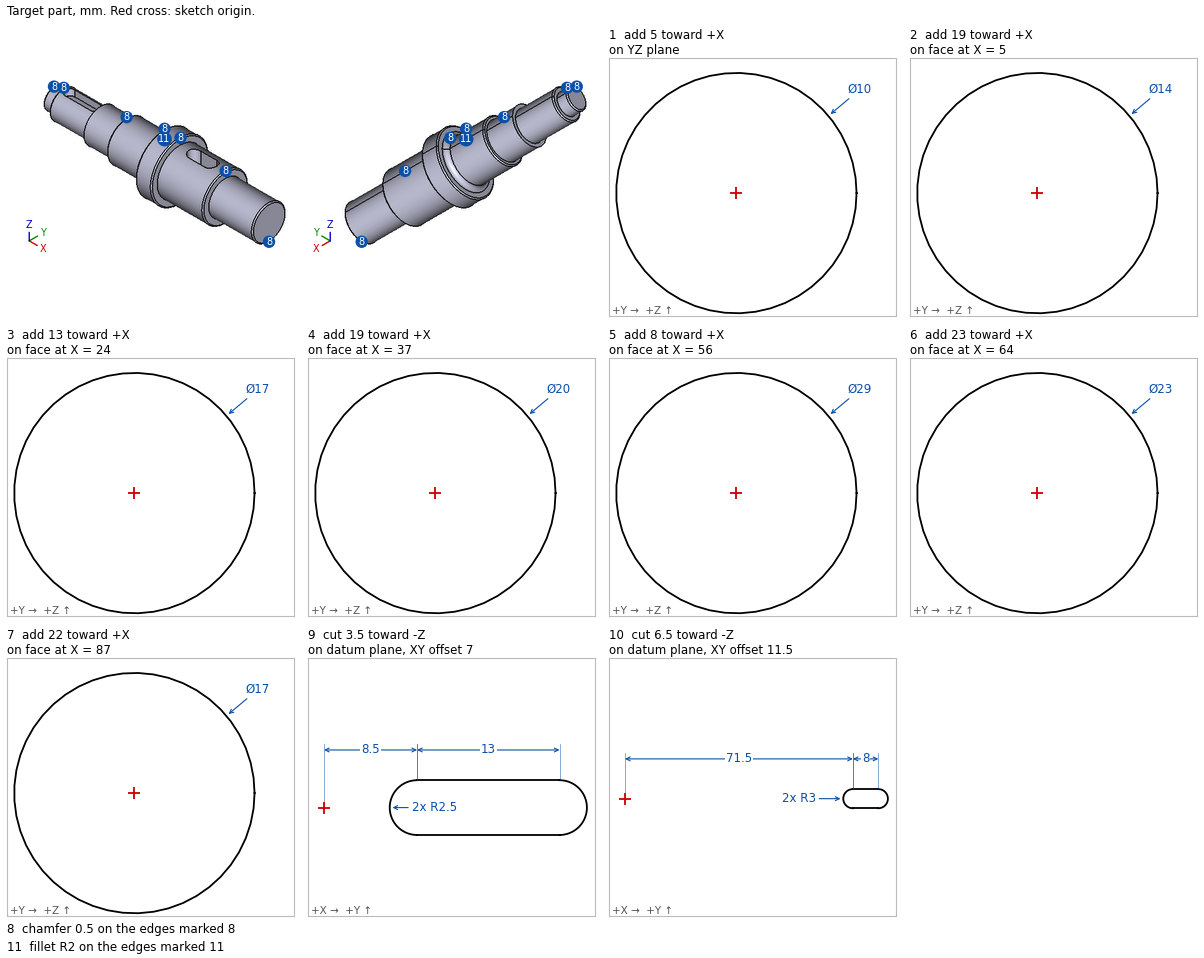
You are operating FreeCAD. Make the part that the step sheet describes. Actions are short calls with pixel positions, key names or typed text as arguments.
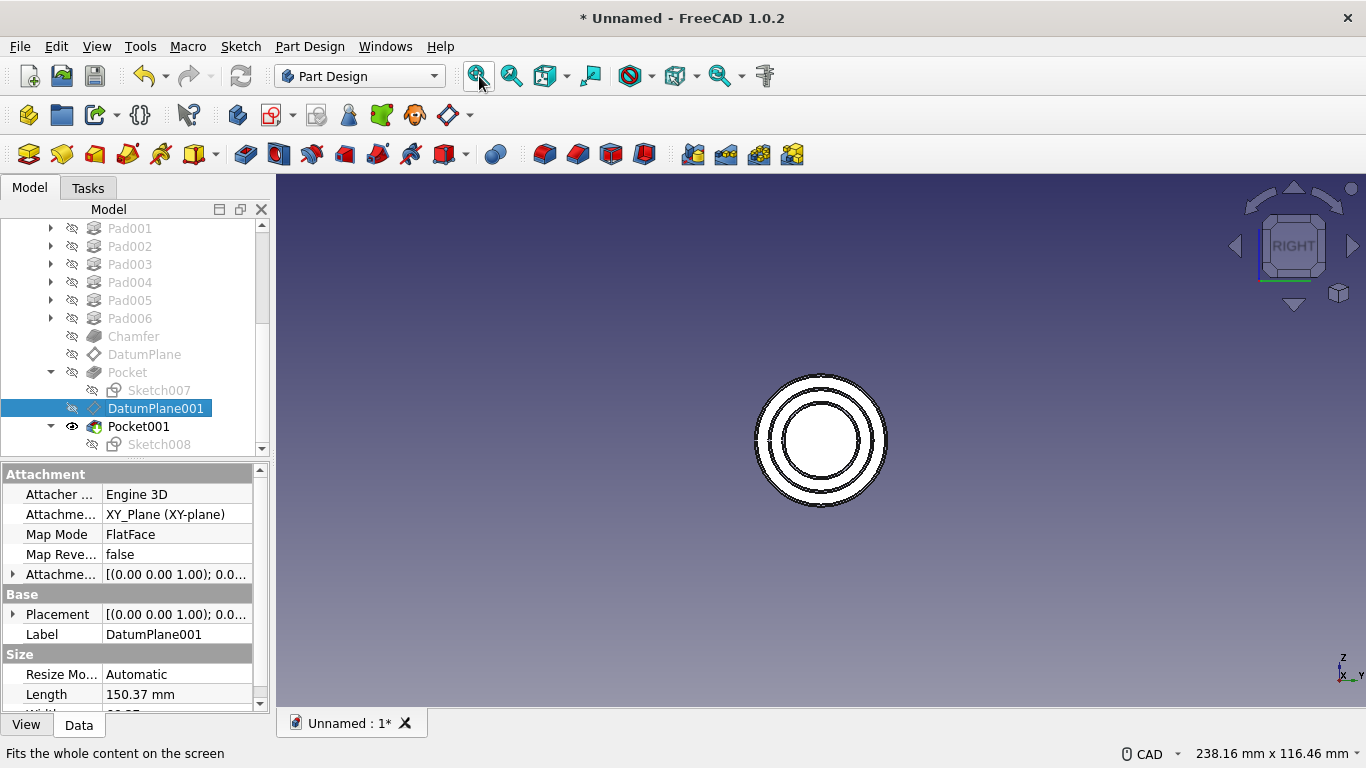
key(5)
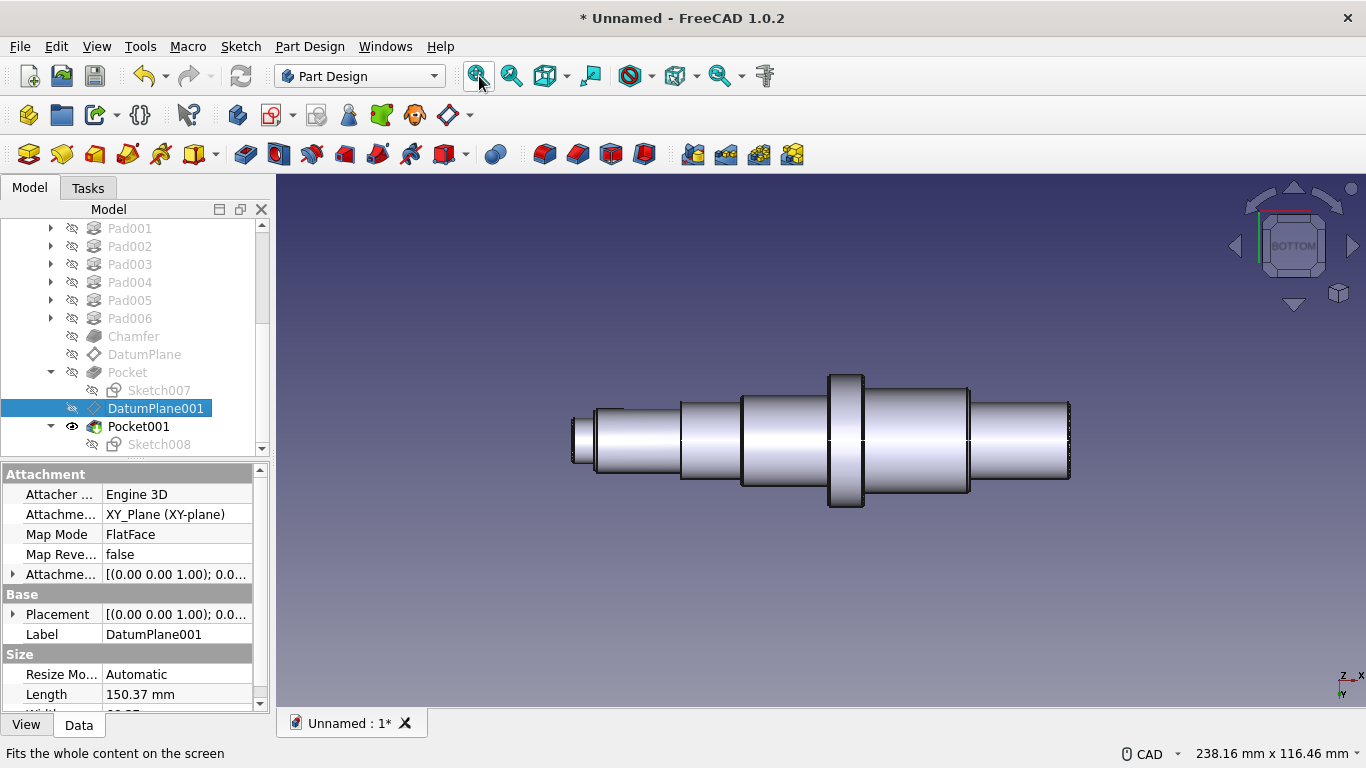
key(4)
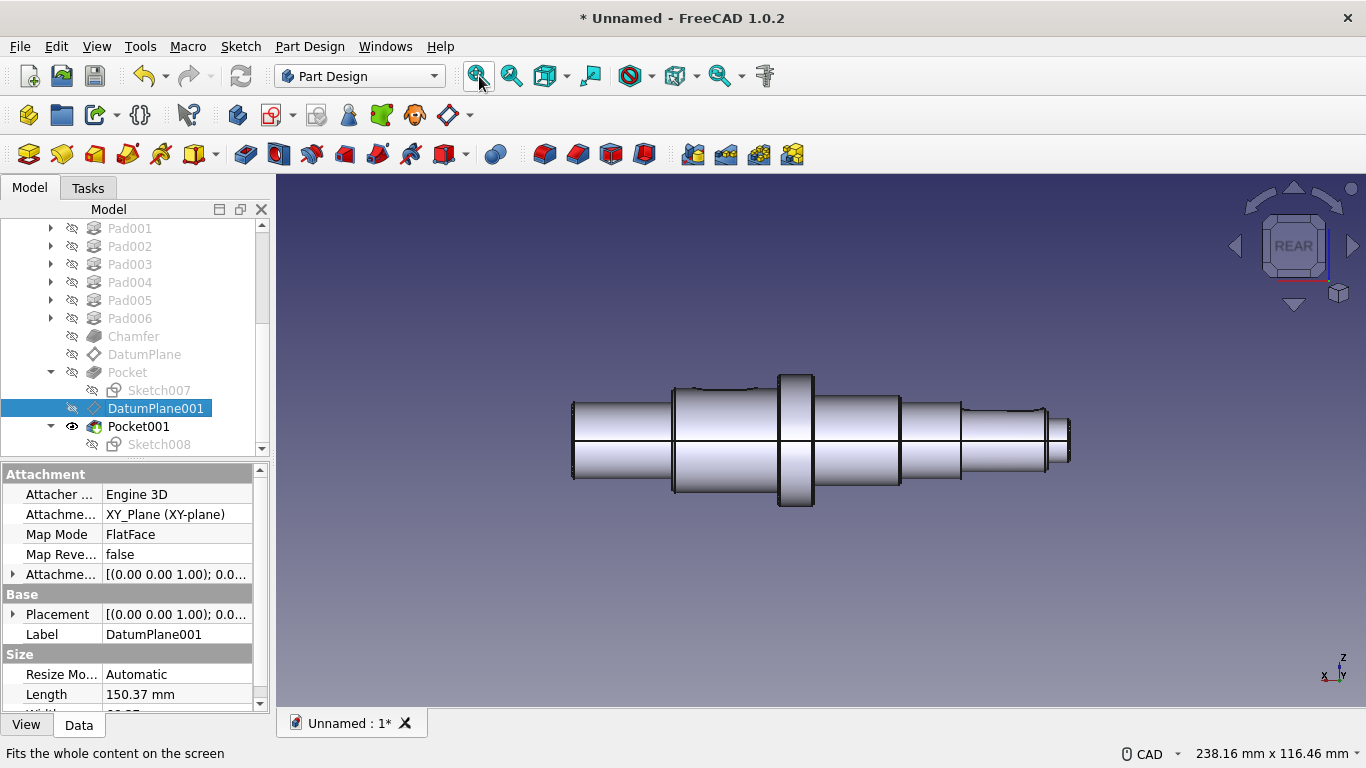
key(6)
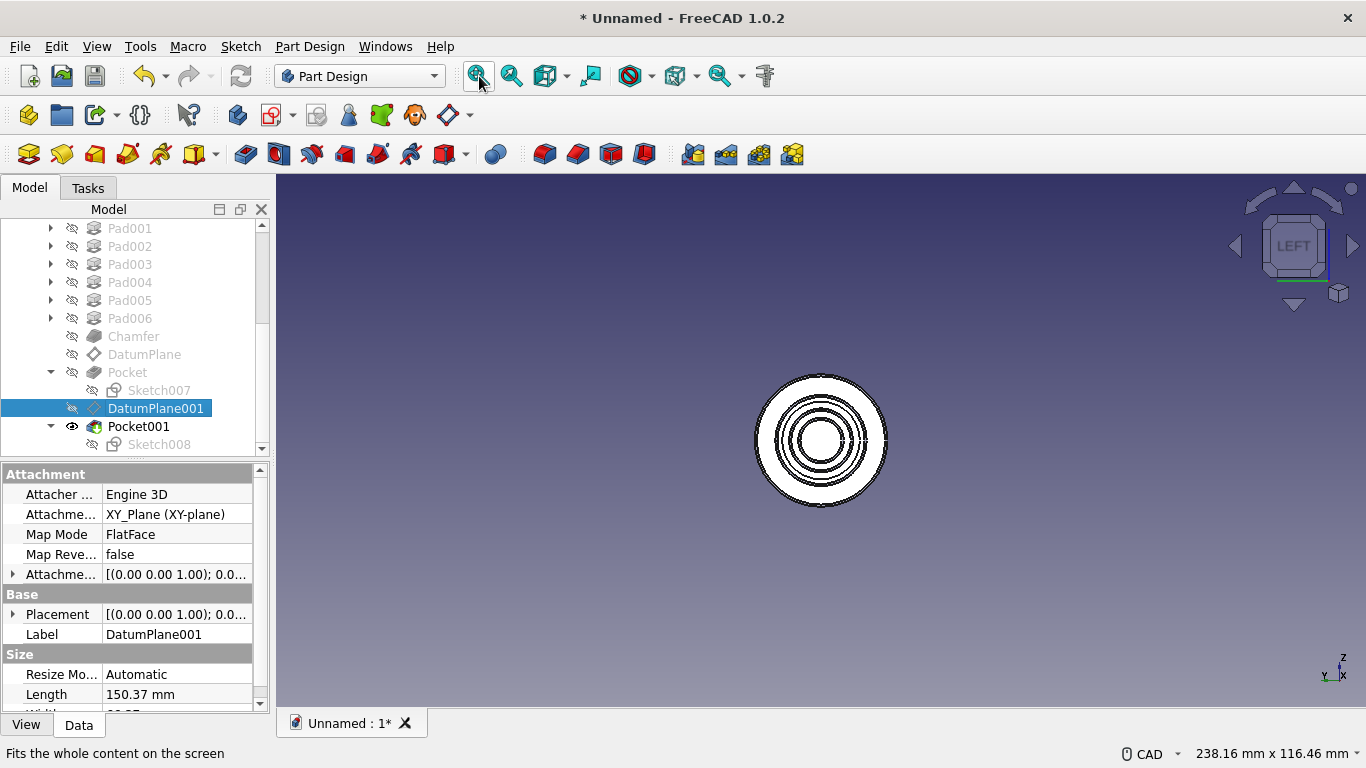
click(479, 76)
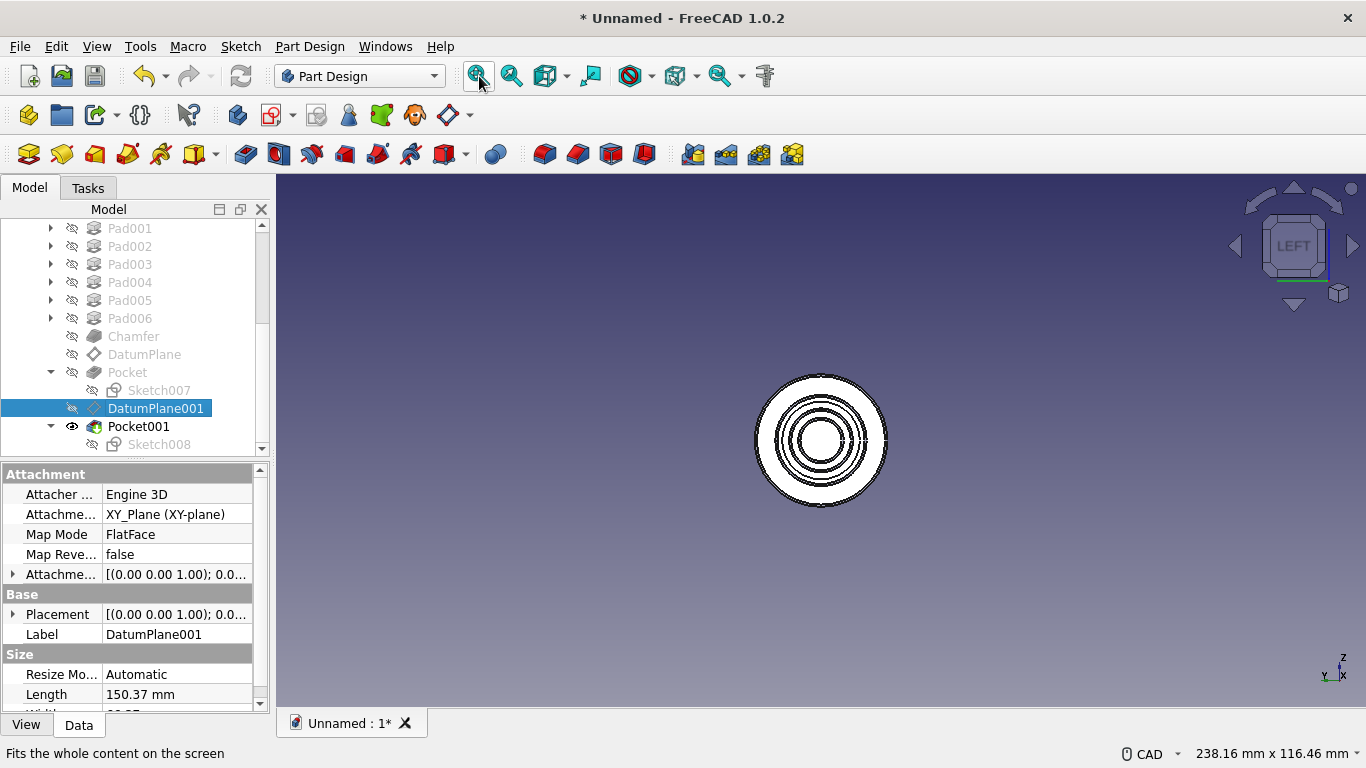
key(v)
key(3)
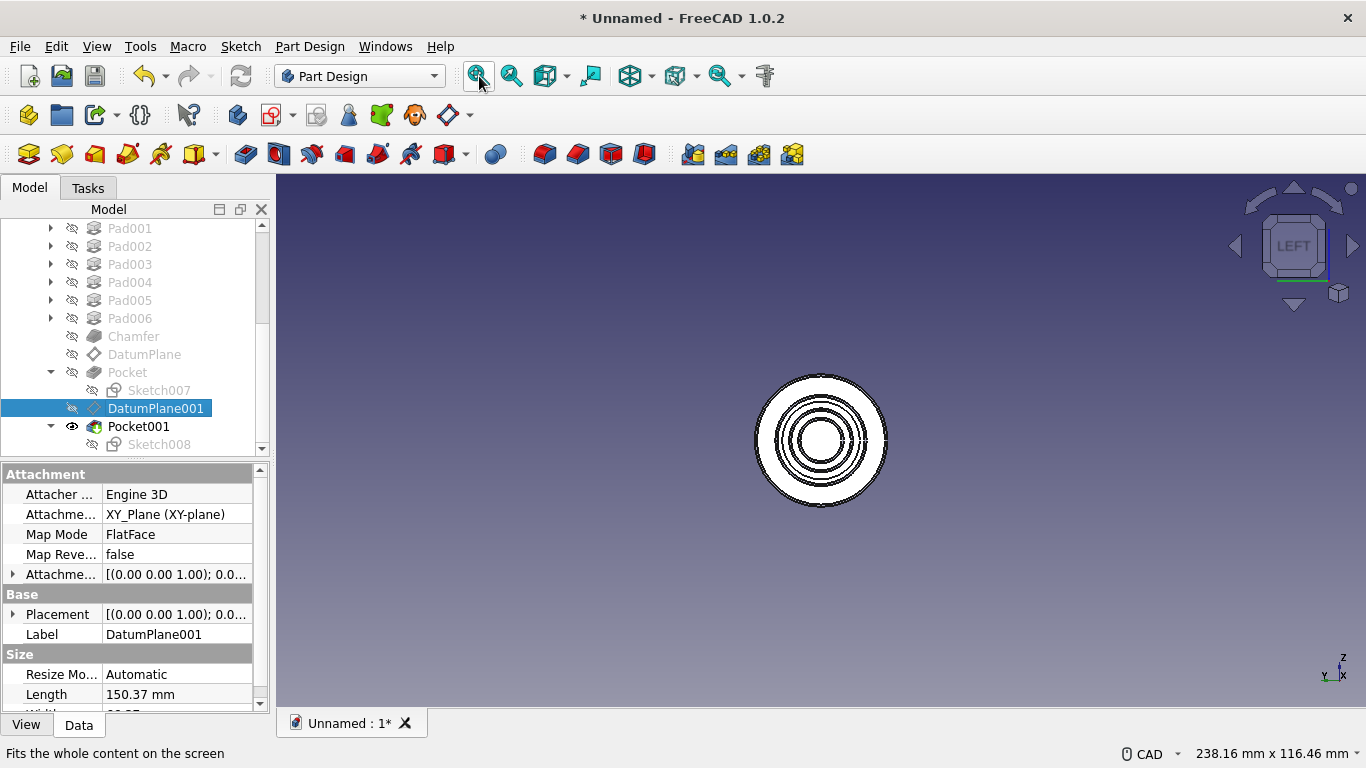
key(0)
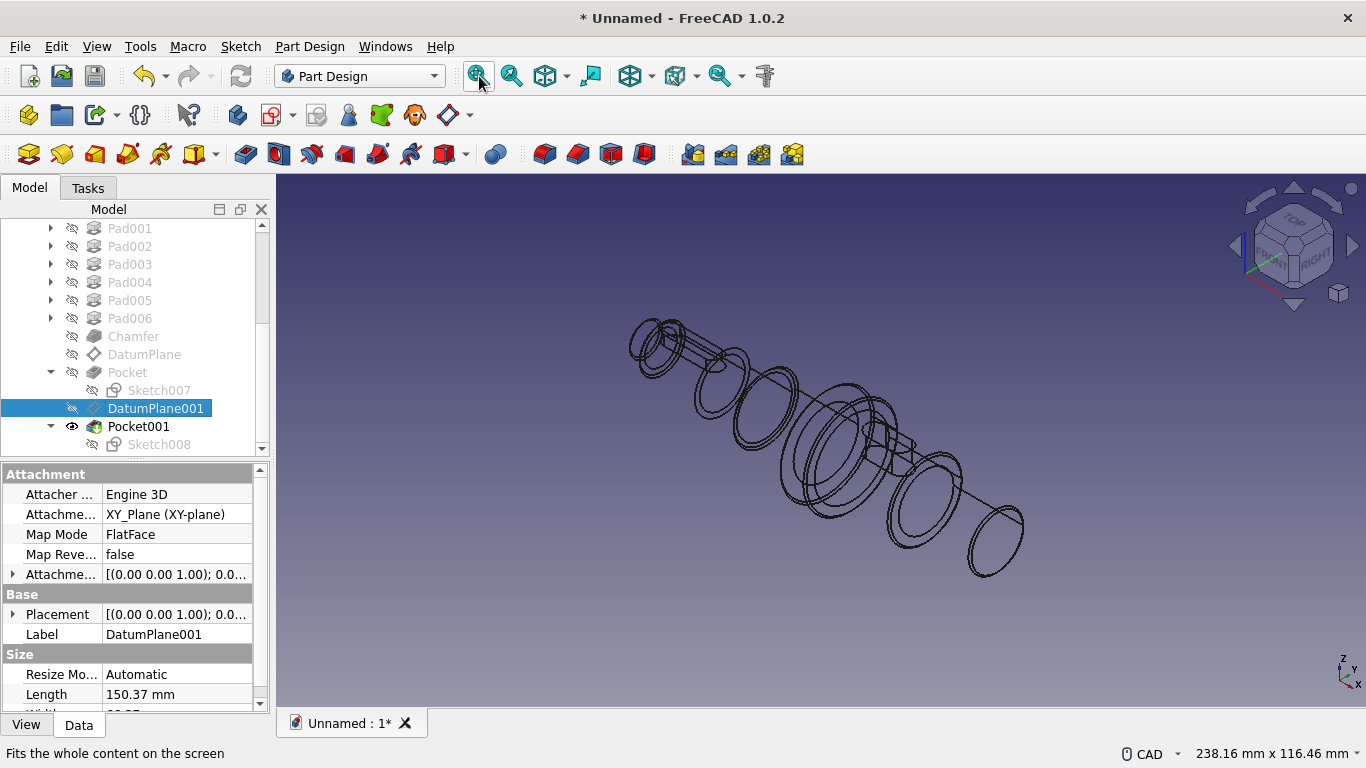
click(793, 461)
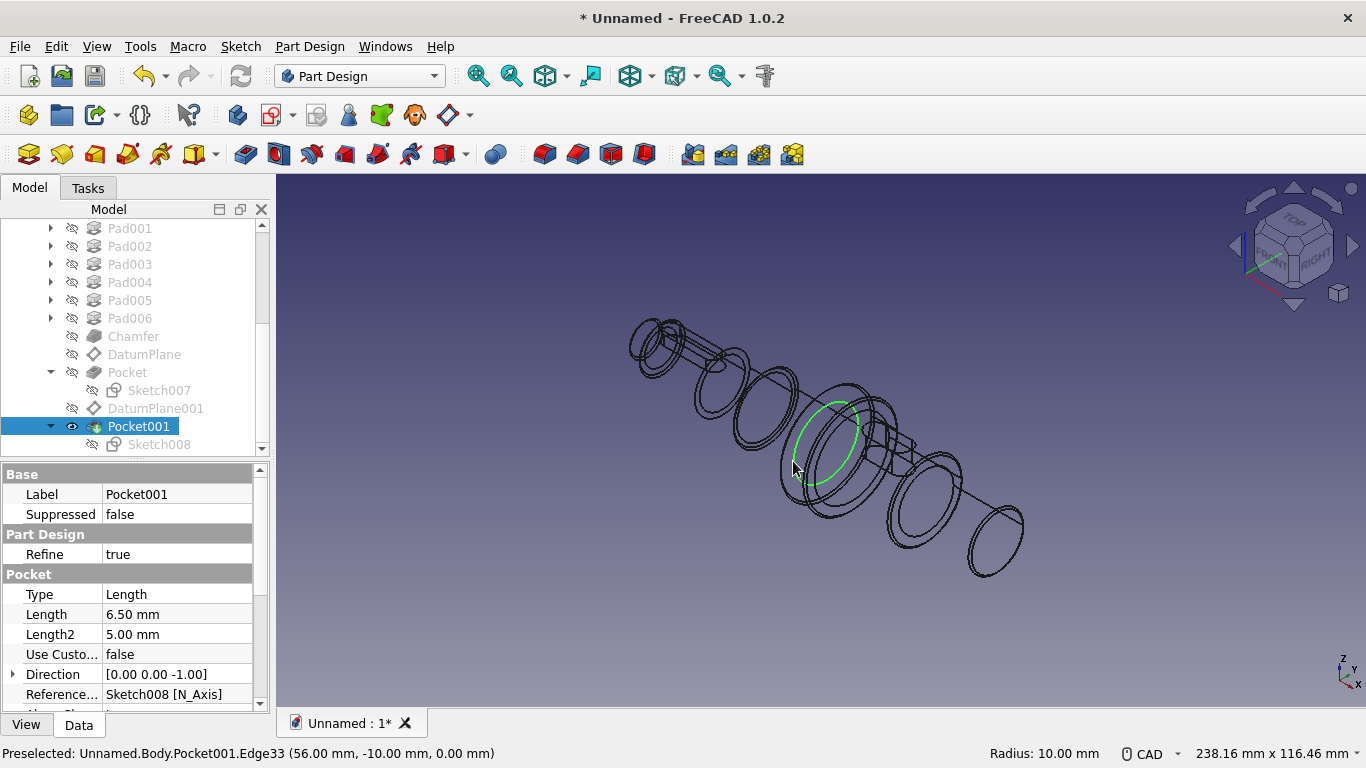
key(v)
key(1)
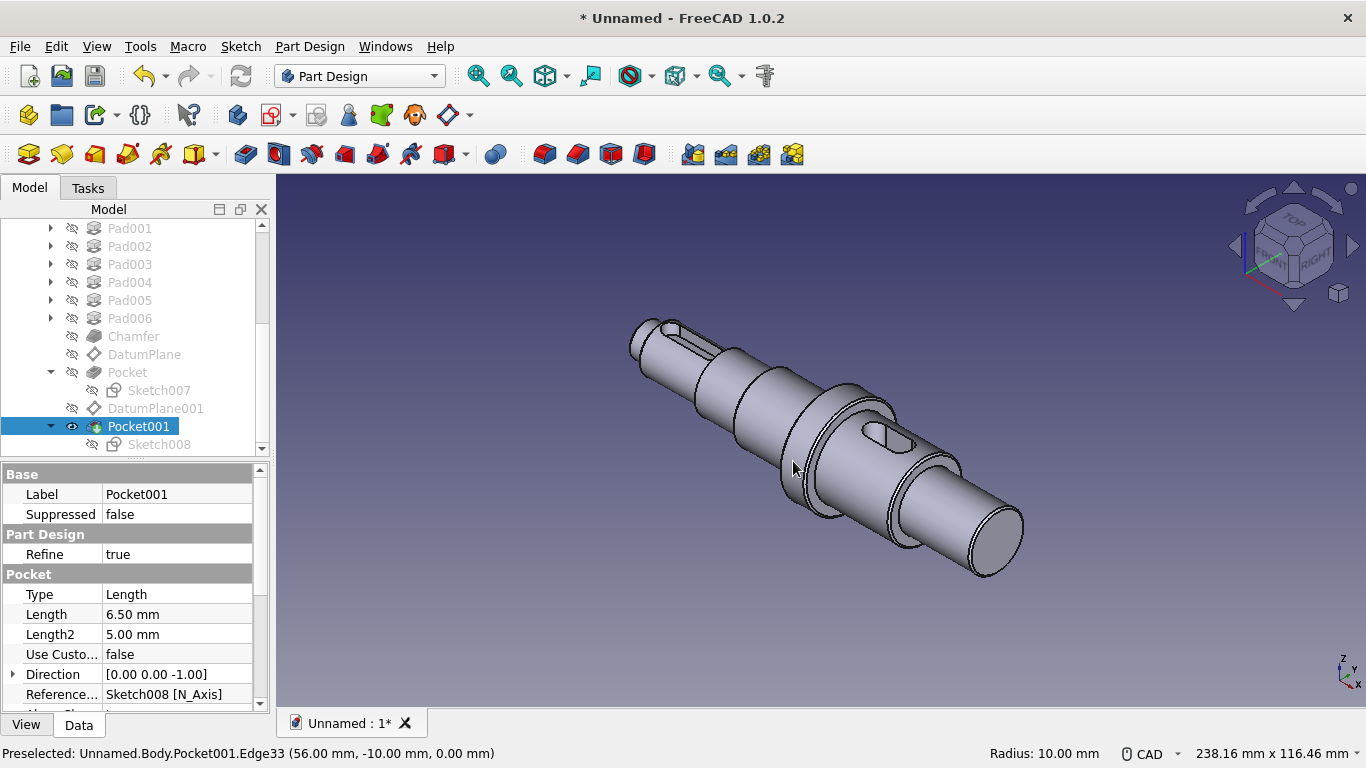
click(545, 154)